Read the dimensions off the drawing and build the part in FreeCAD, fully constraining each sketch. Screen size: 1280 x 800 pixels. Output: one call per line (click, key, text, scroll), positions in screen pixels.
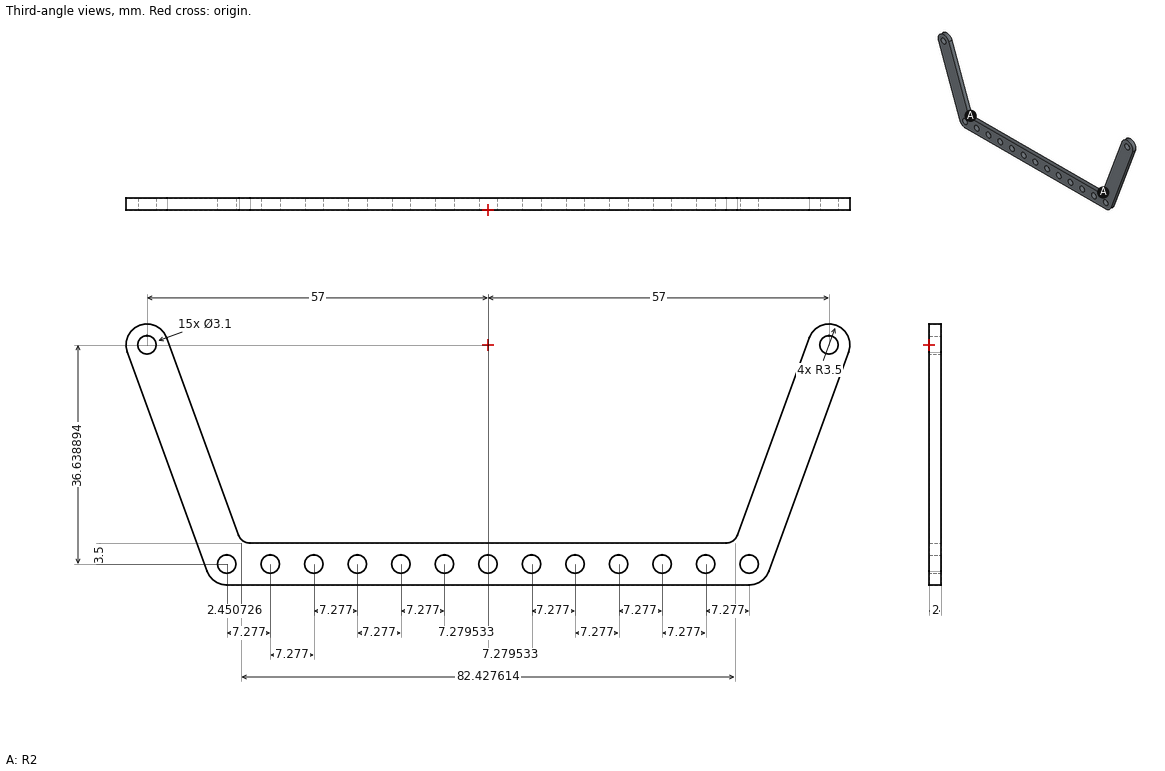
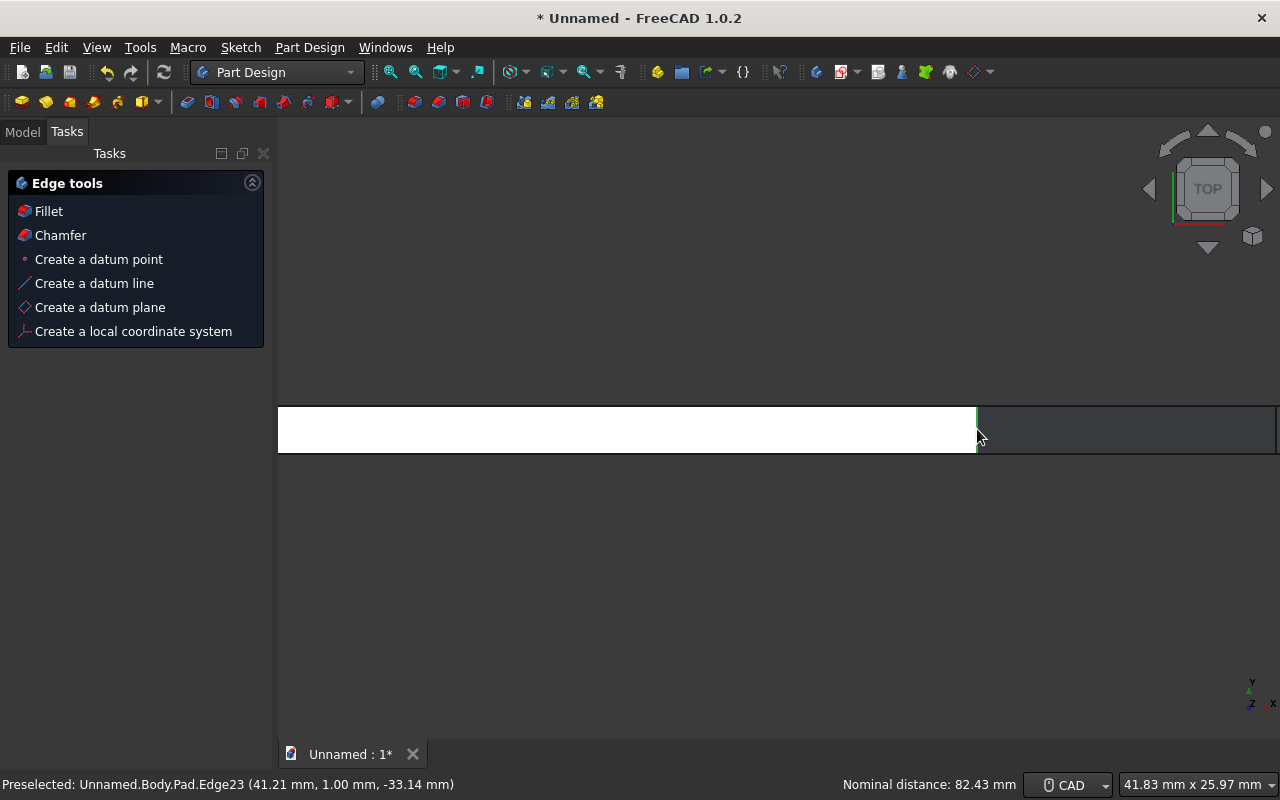
click(416, 102)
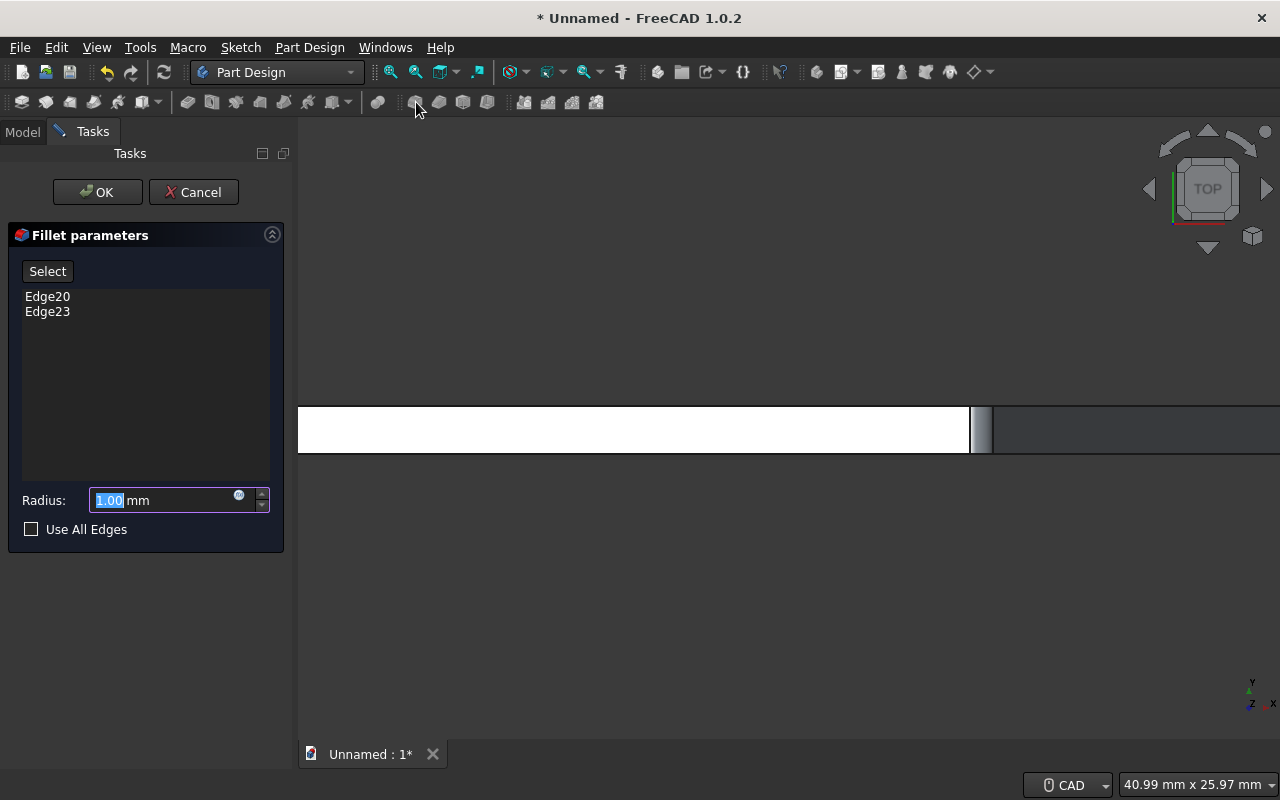
text(2)
key(Tab)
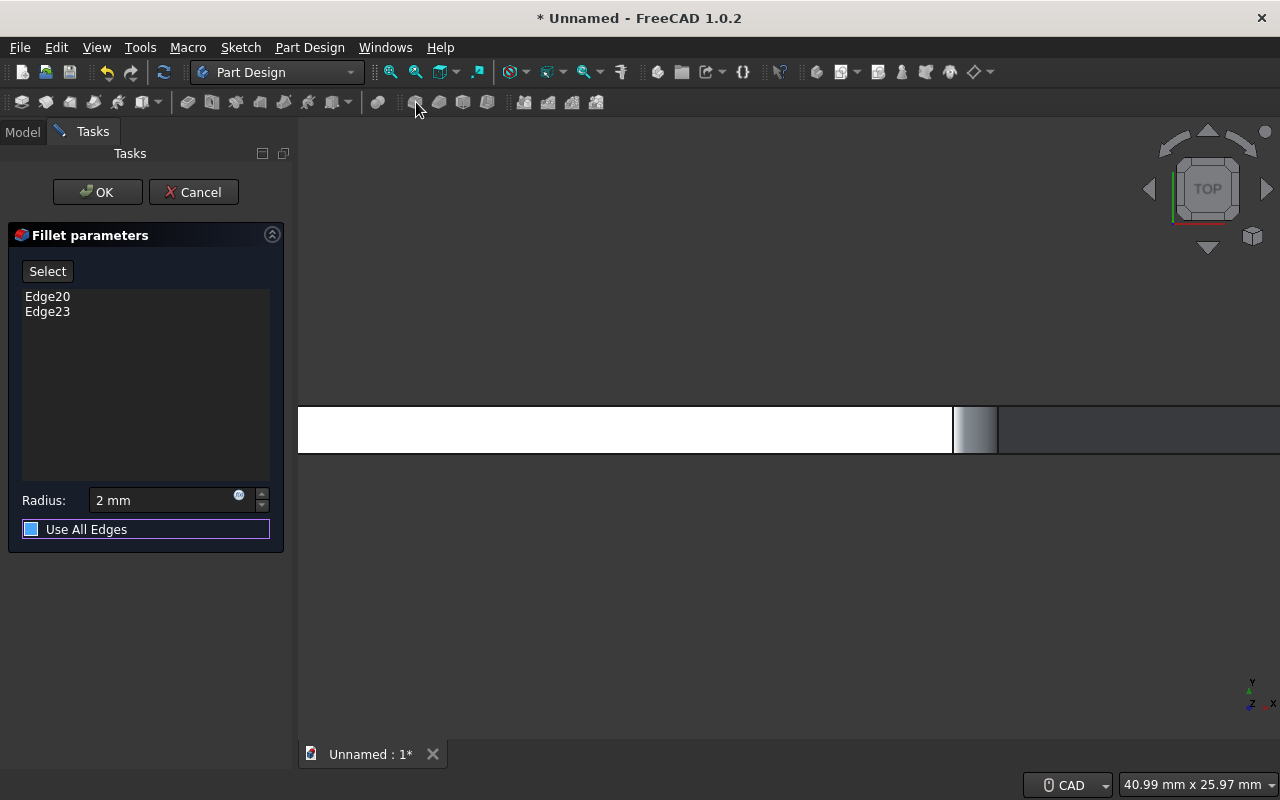
click(98, 192)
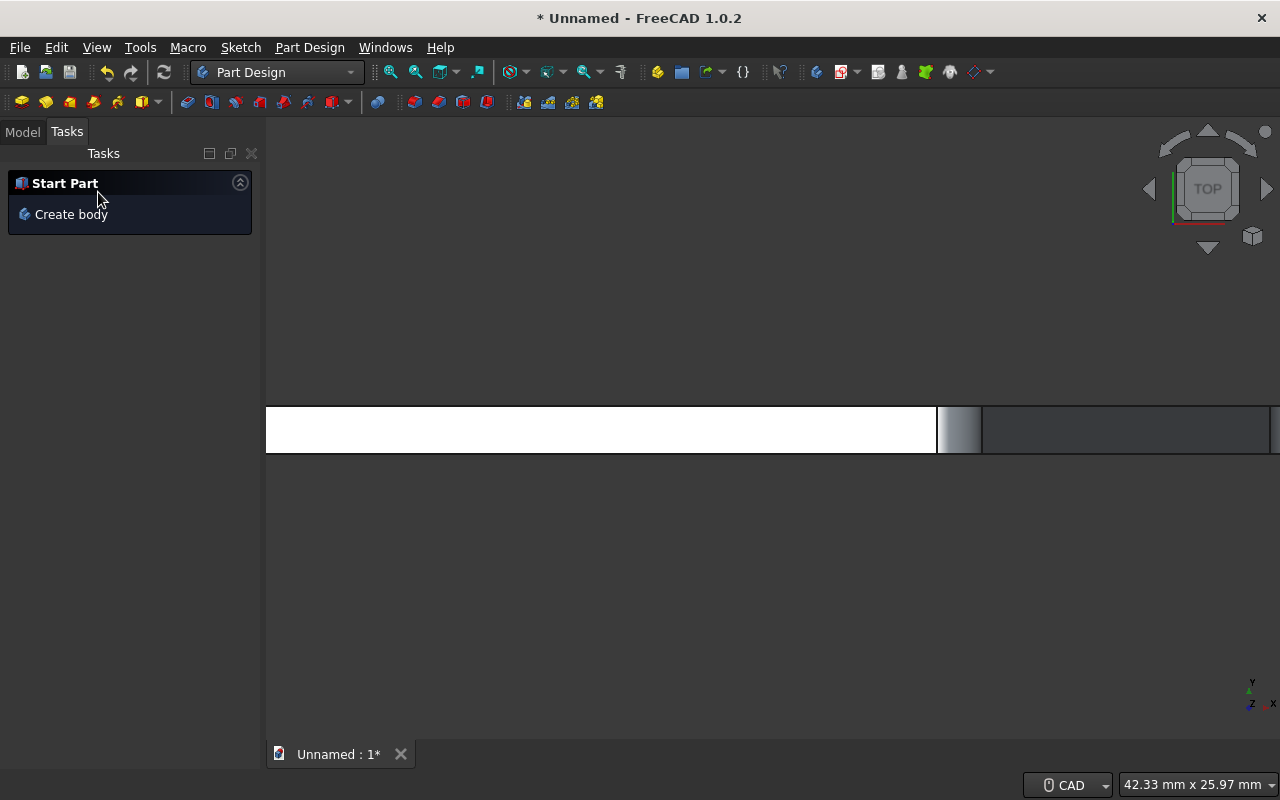
key(0)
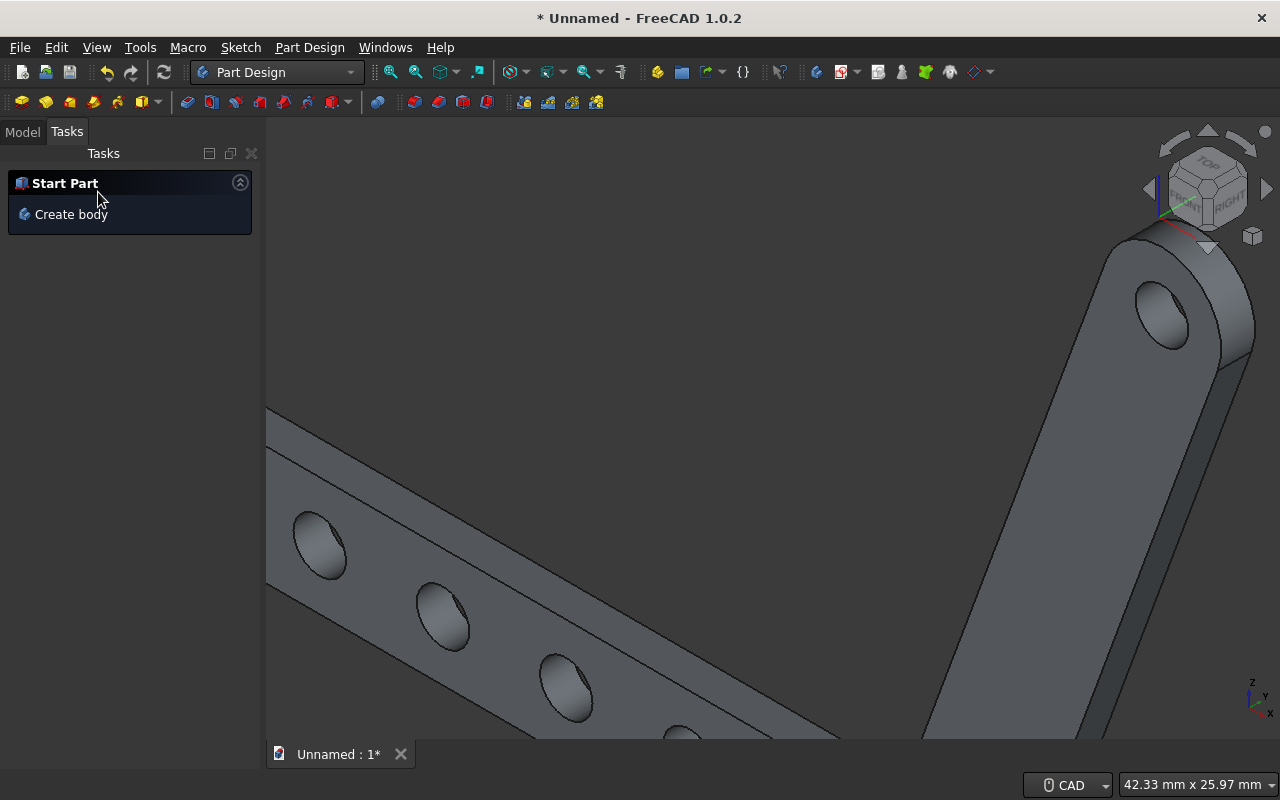
key(v)
key(f)